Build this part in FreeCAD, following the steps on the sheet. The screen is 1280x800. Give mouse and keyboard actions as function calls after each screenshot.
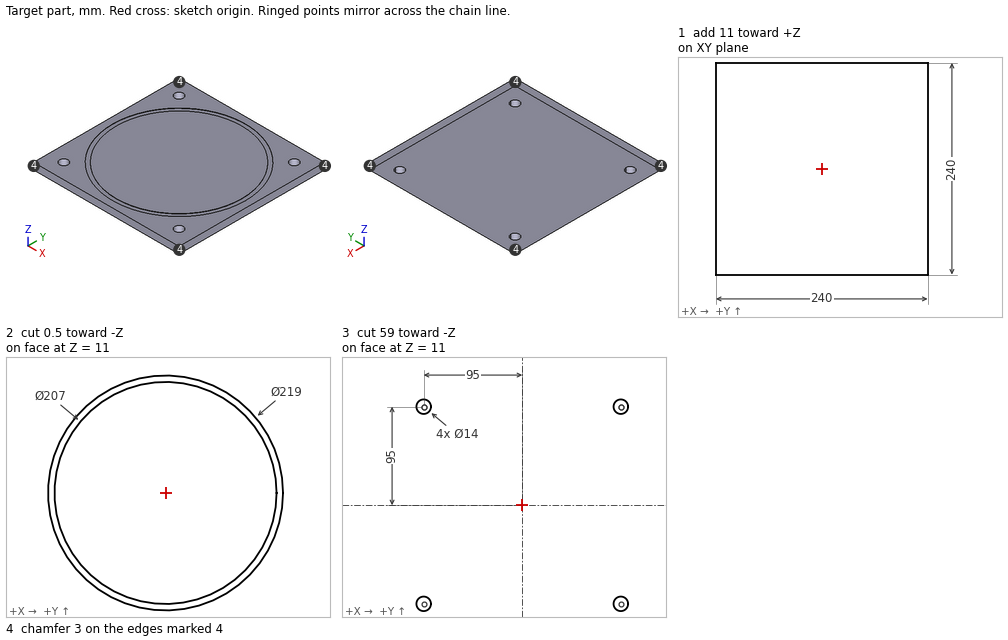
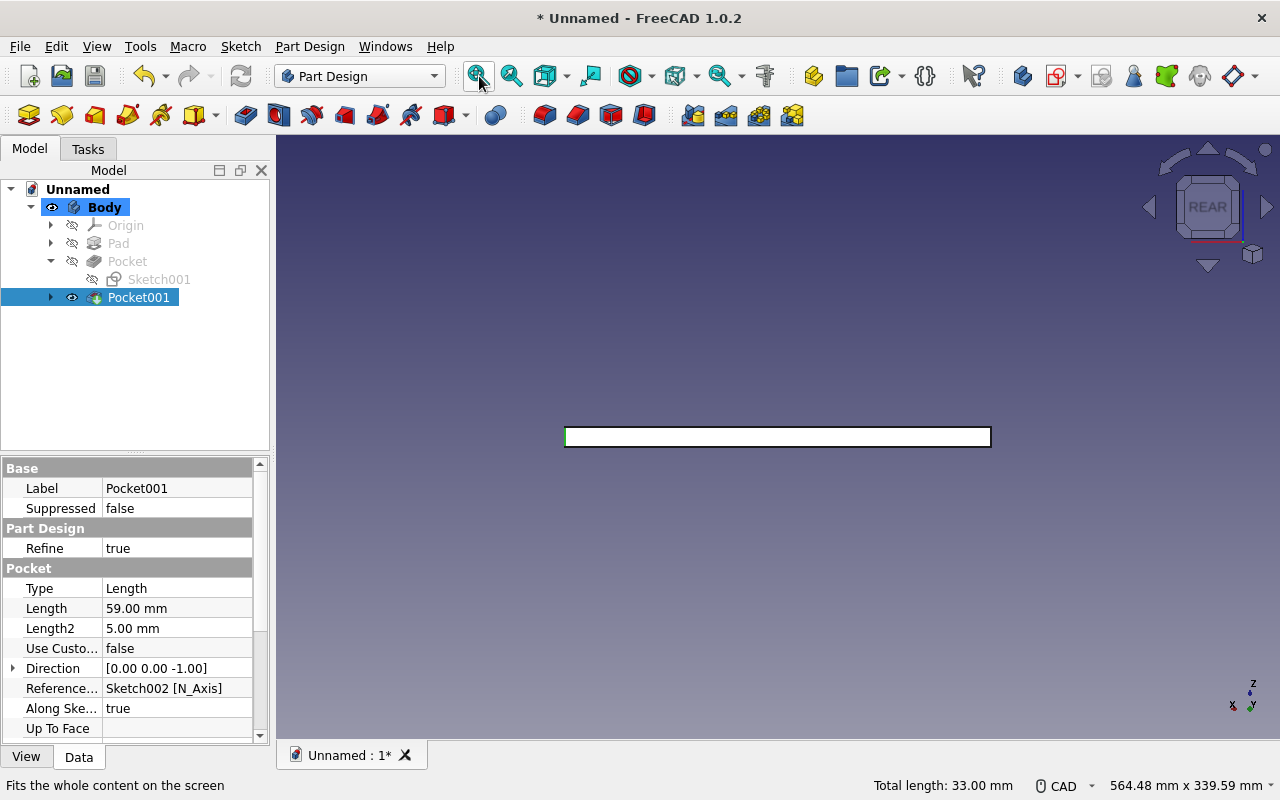
click(991, 436, ctrl)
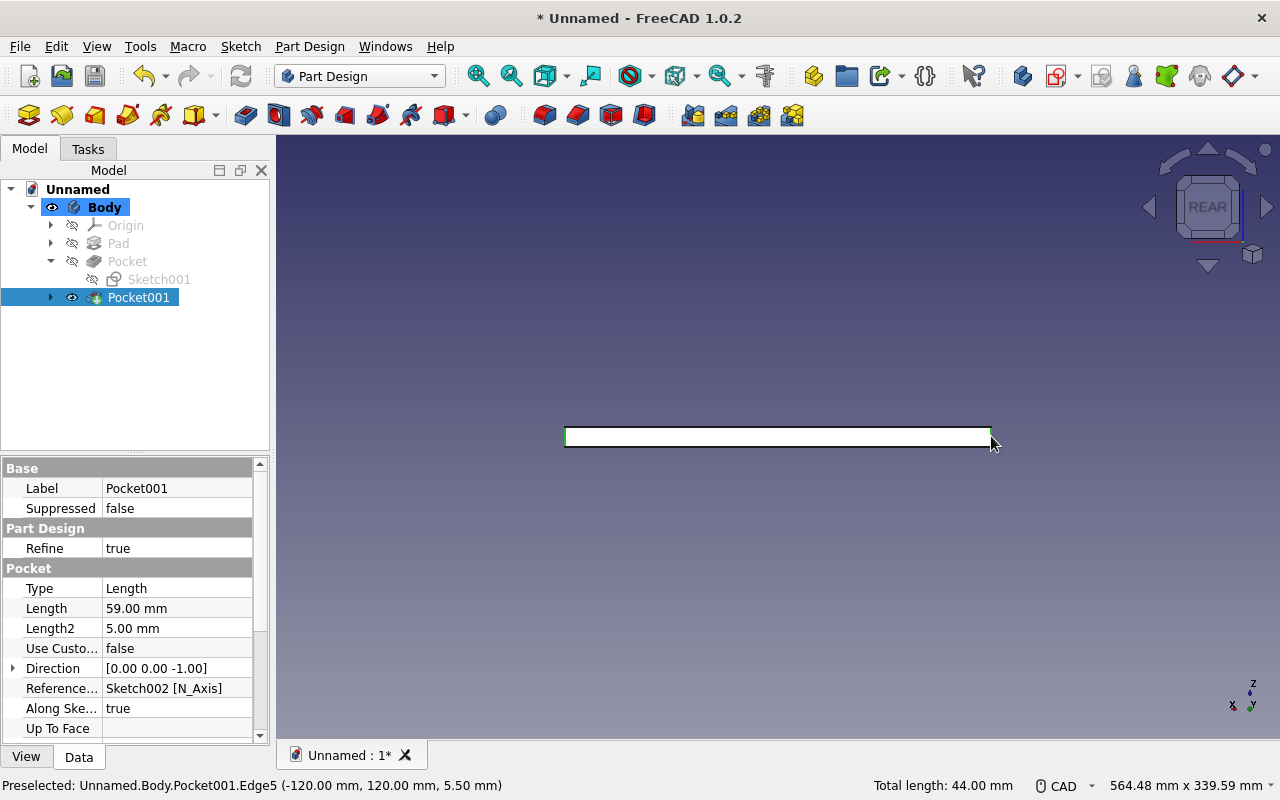
click(578, 116)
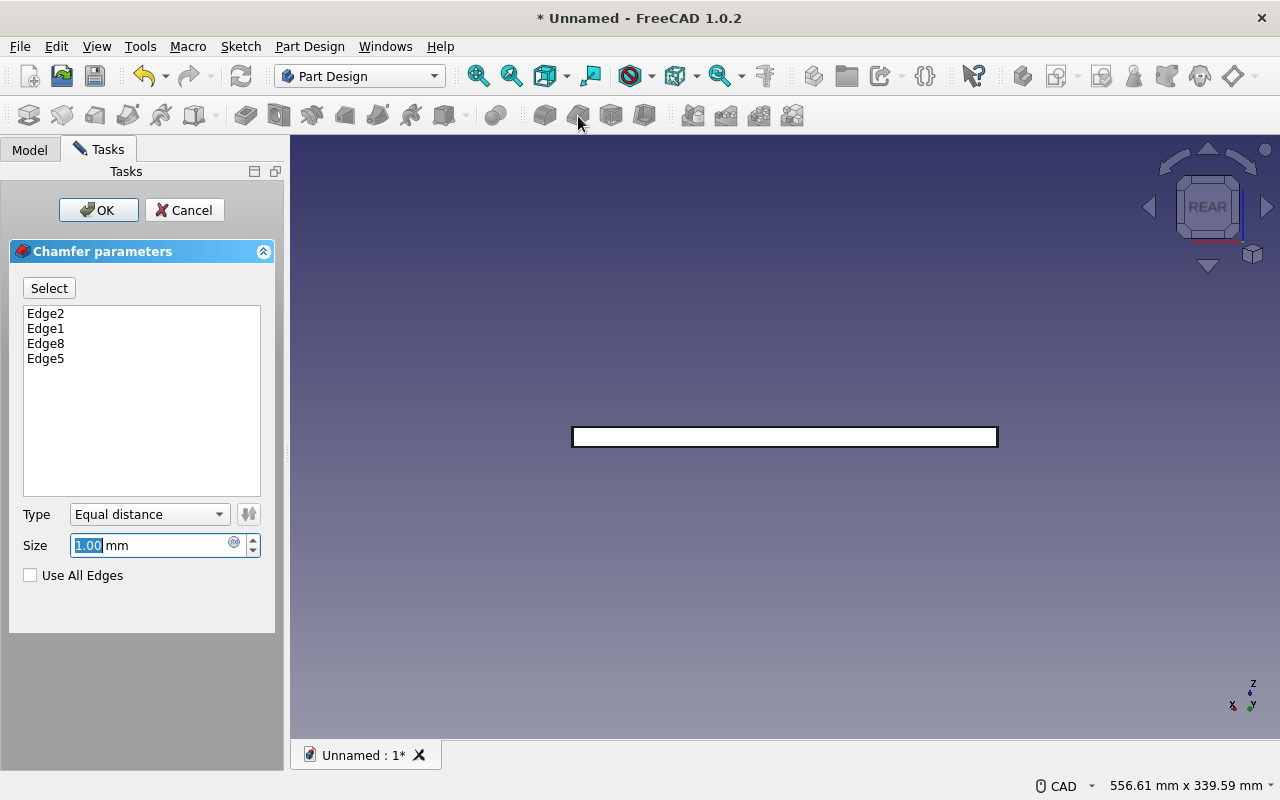
text(3)
key(Tab)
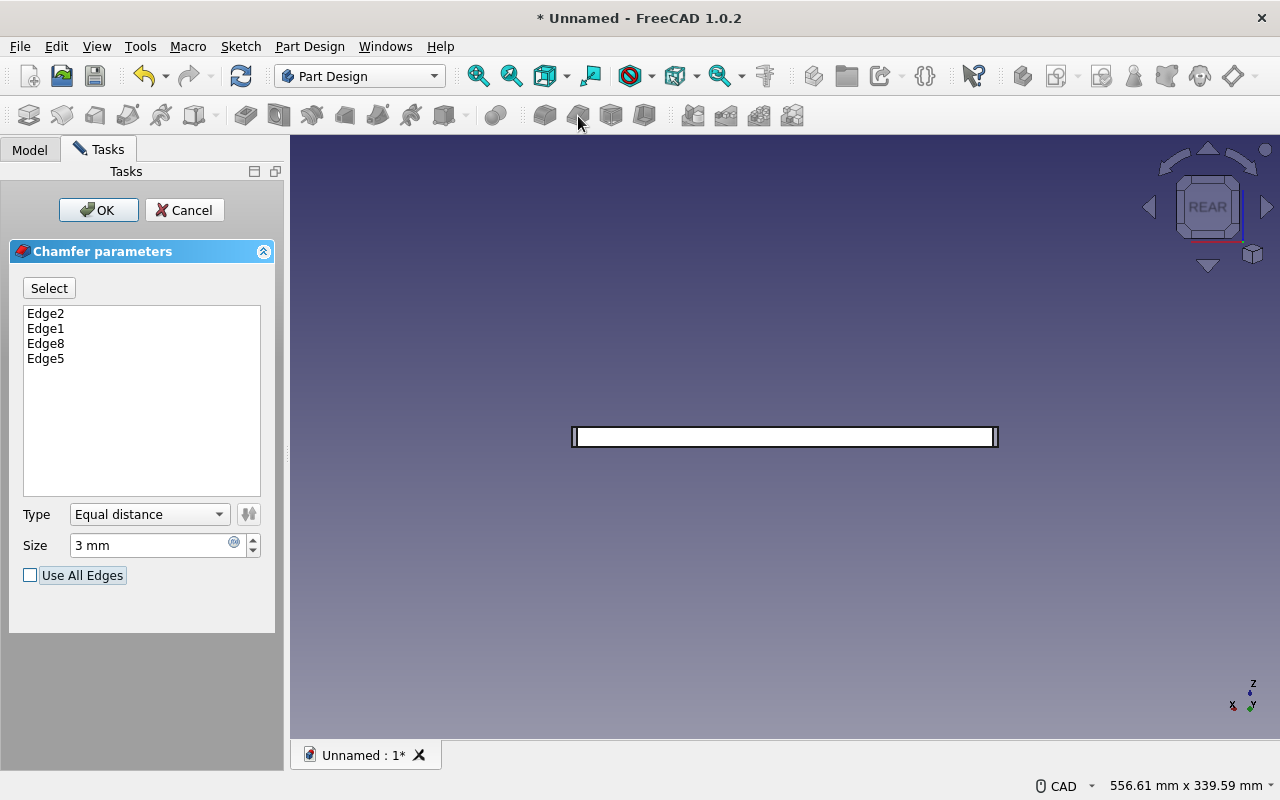
click(99, 210)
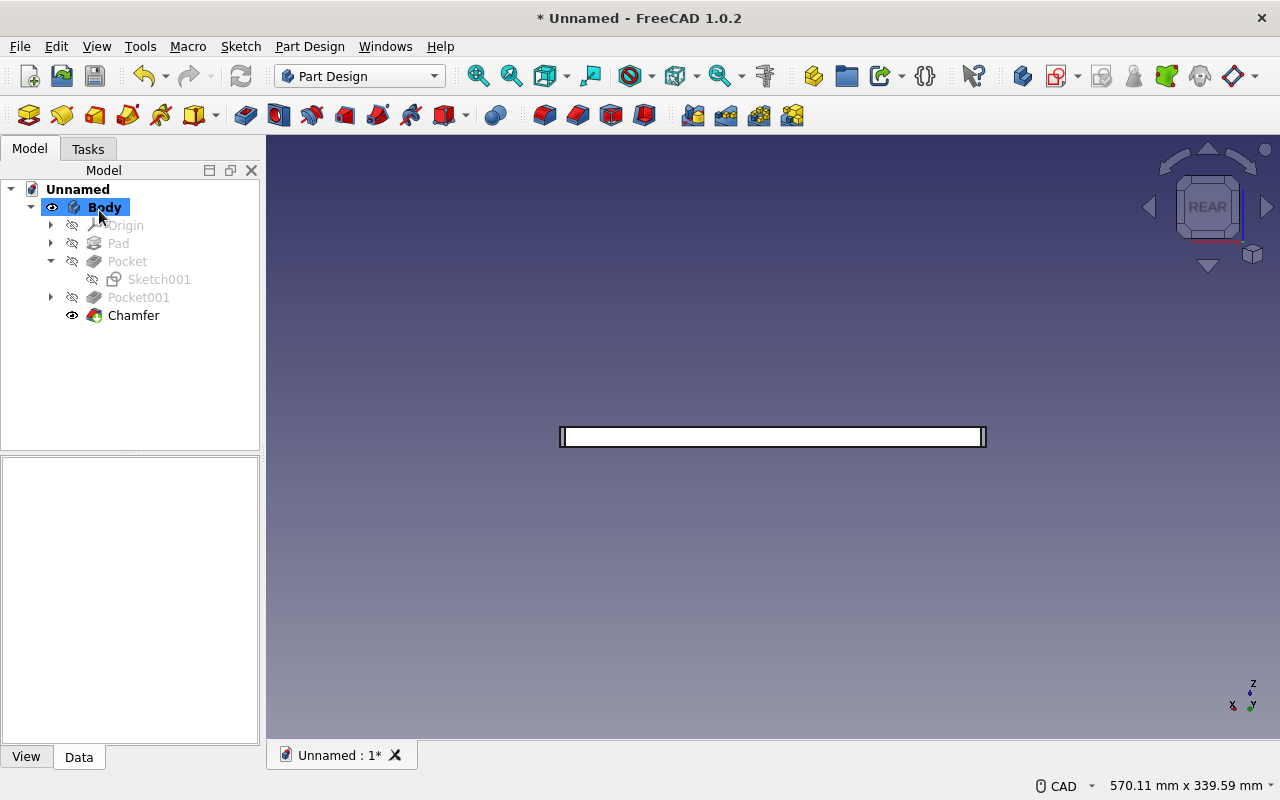
key(0)